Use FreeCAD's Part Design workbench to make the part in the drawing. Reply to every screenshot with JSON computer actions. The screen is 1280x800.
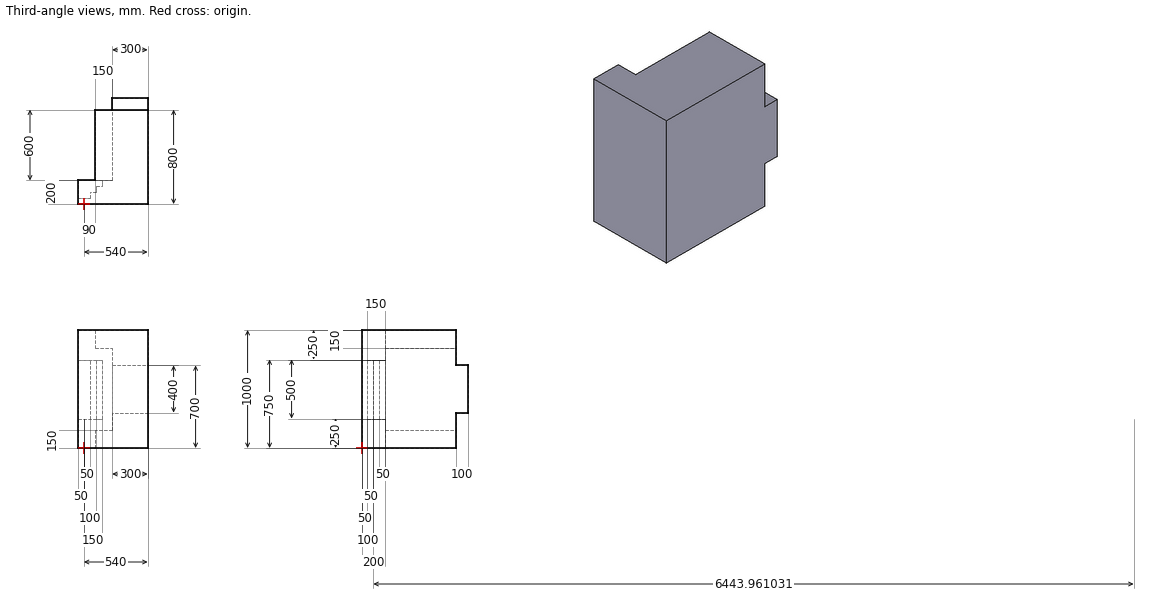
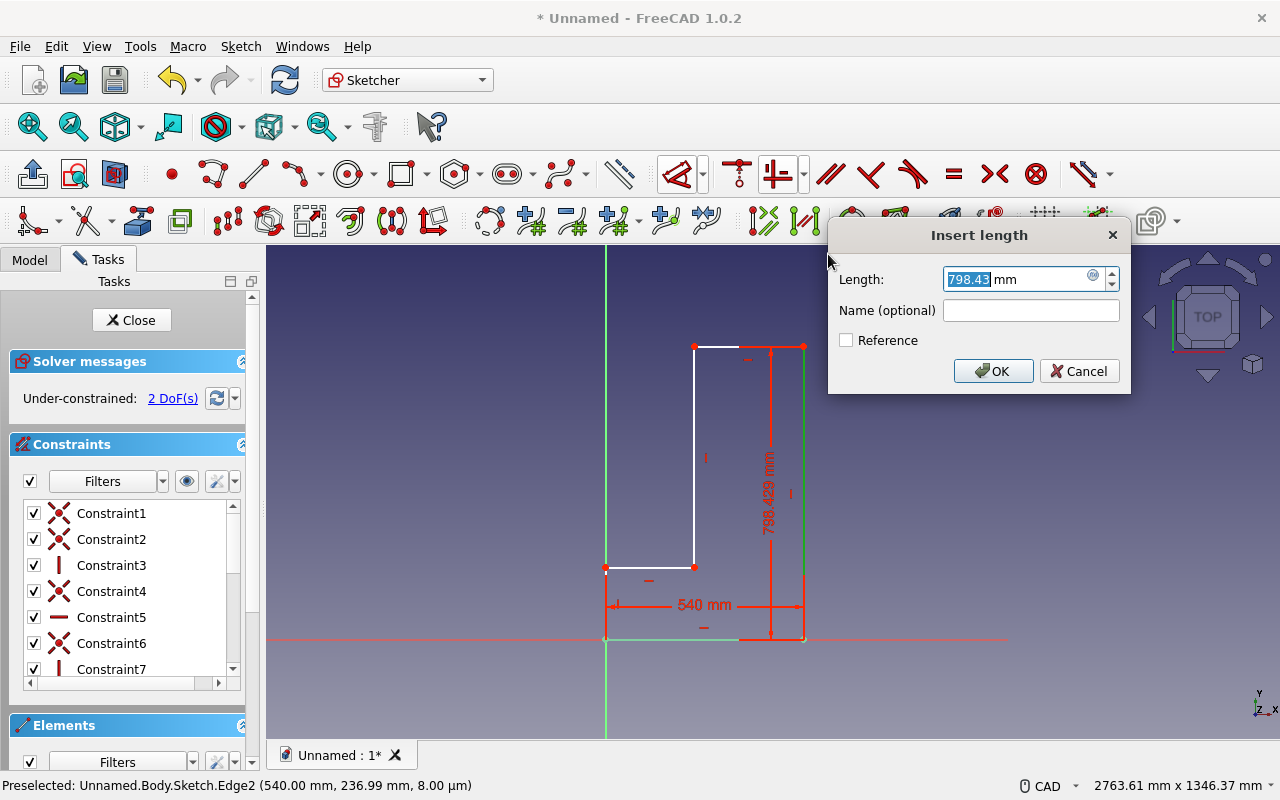
{"action": "type", "text": "800"}
{"action": "key", "text": "Return"}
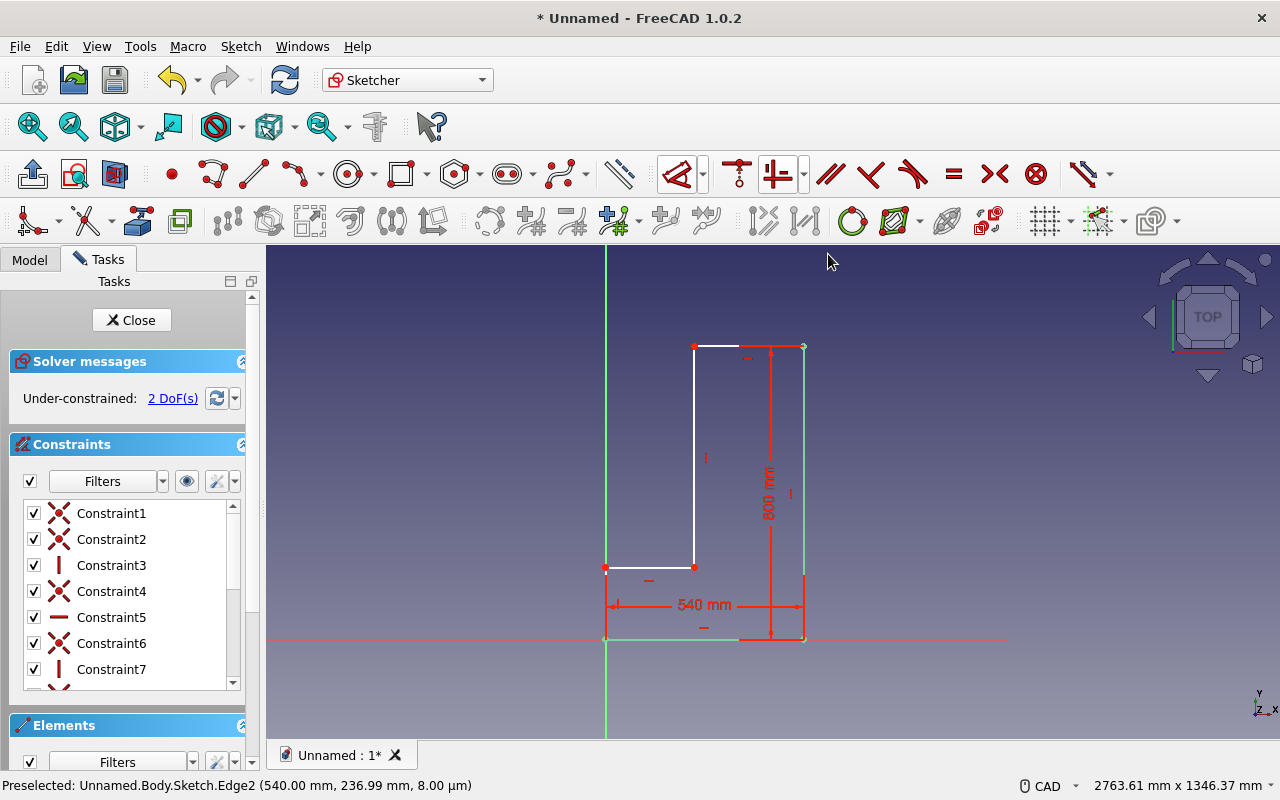
{"action": "left_click", "coordinate": [771, 346]}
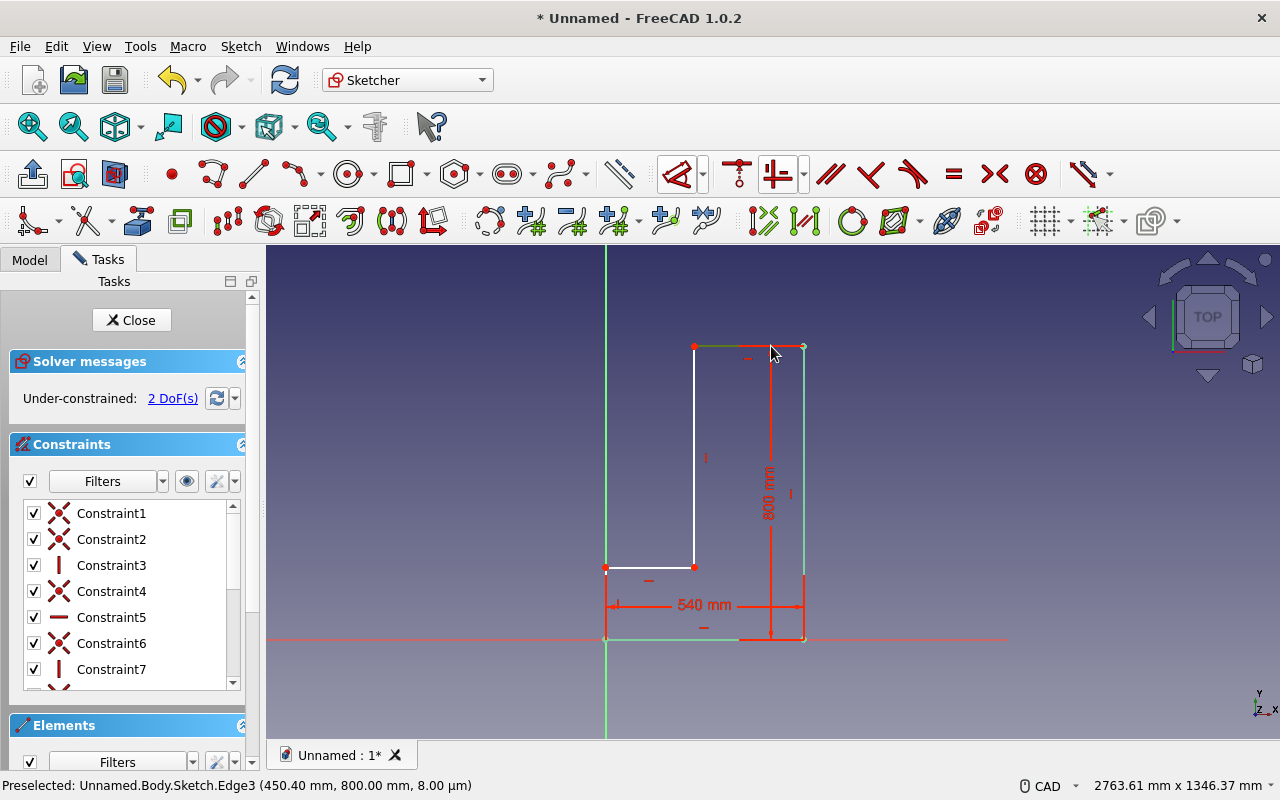
{"action": "key", "text": "l"}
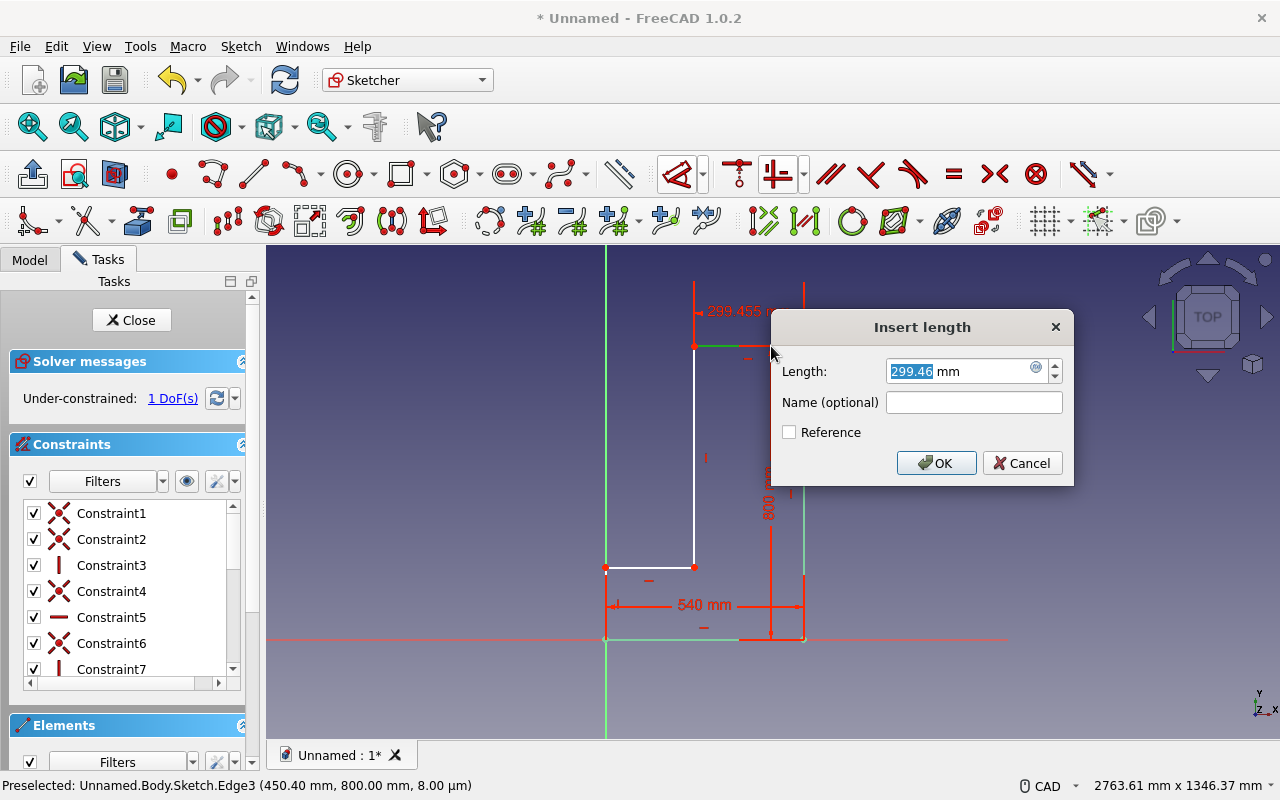
{"action": "type", "text": "300"}
{"action": "key", "text": "Return"}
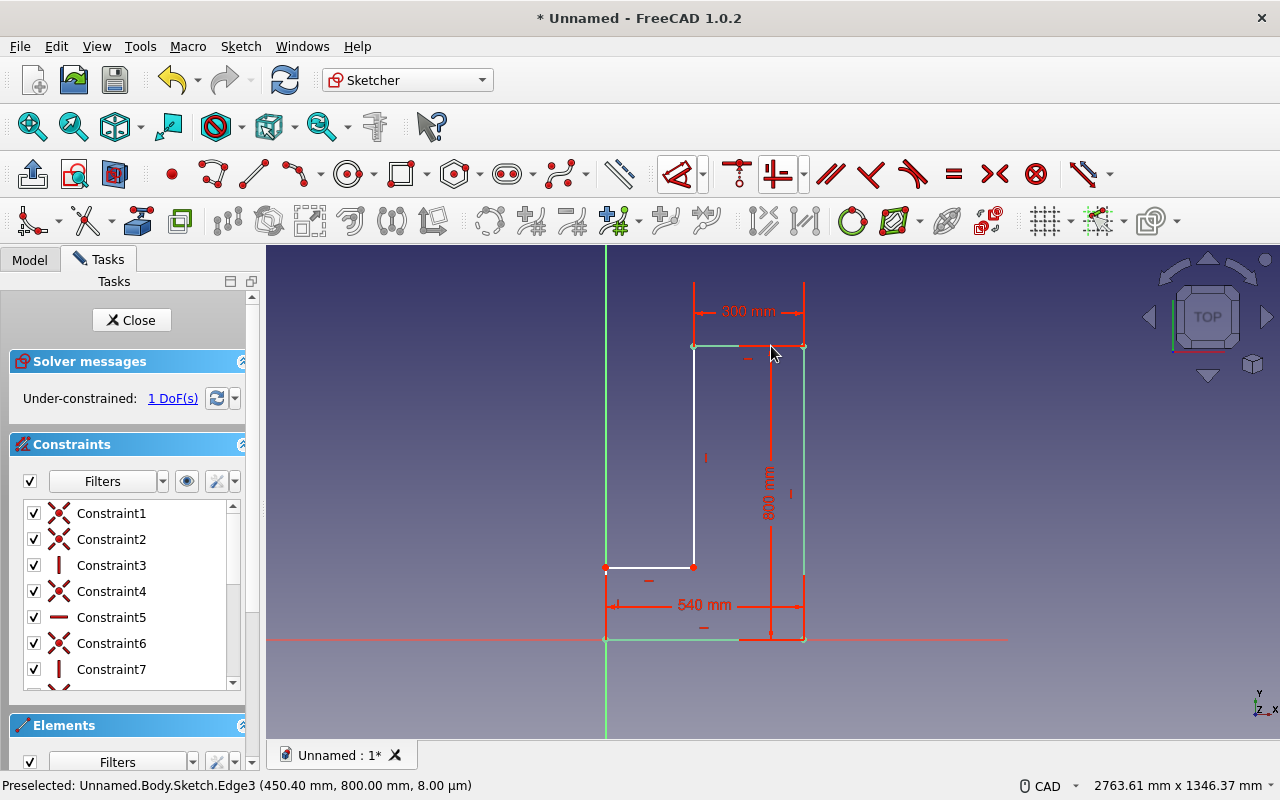
{"action": "left_click", "coordinate": [694, 413]}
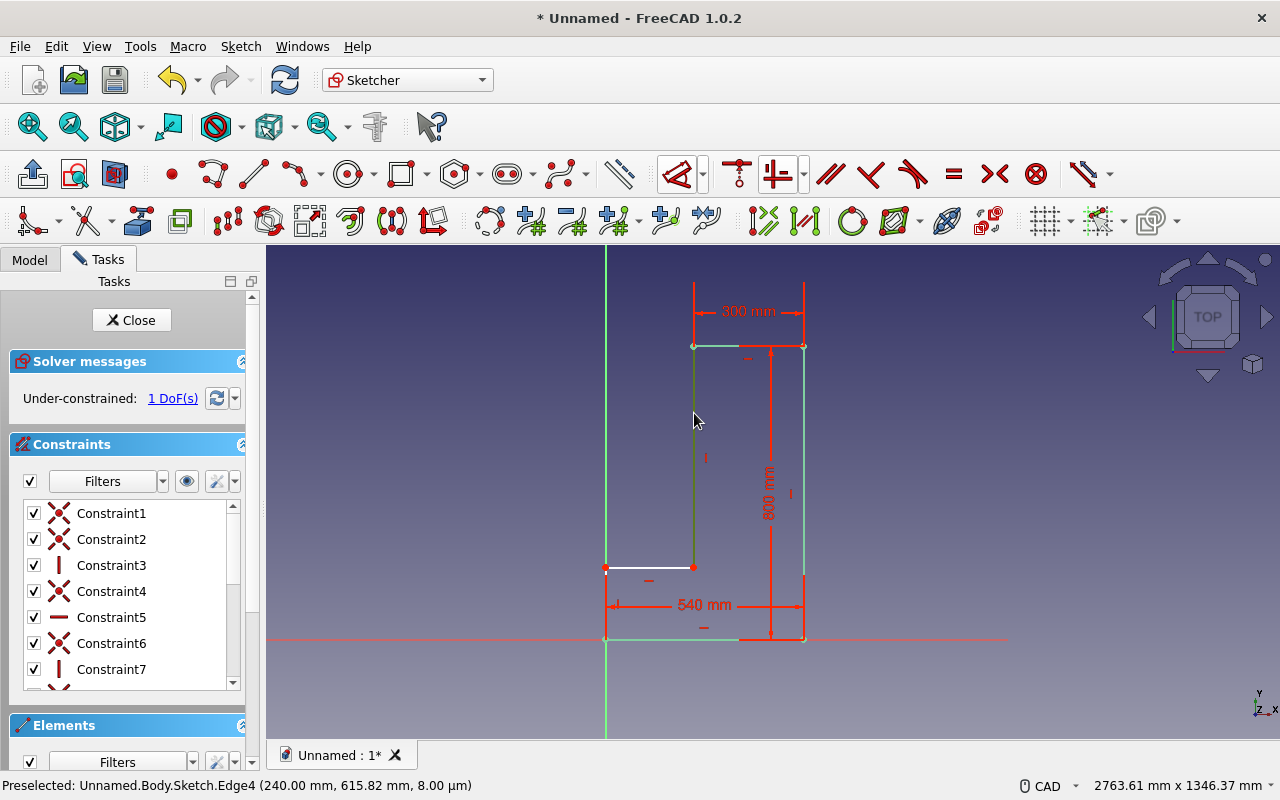
{"action": "key", "text": "i"}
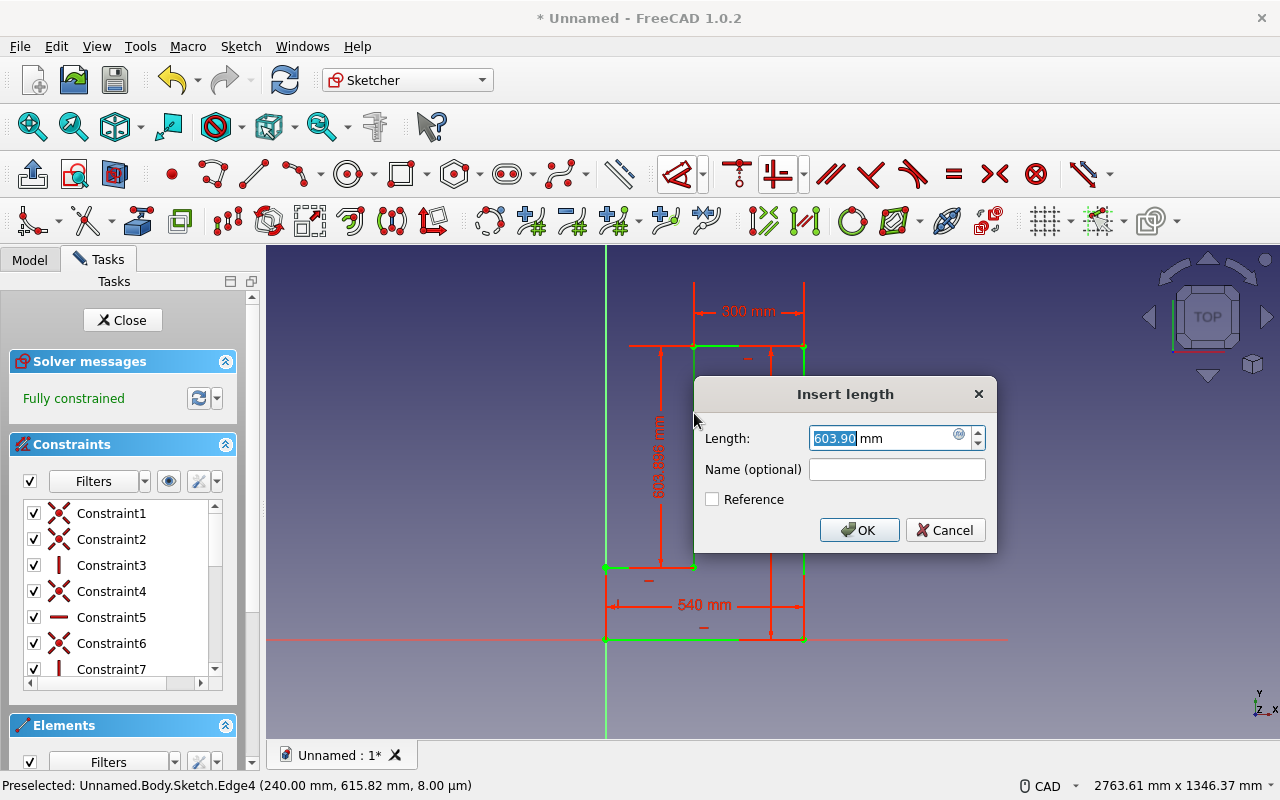
{"action": "type", "text": "600"}
{"action": "key", "text": "Return"}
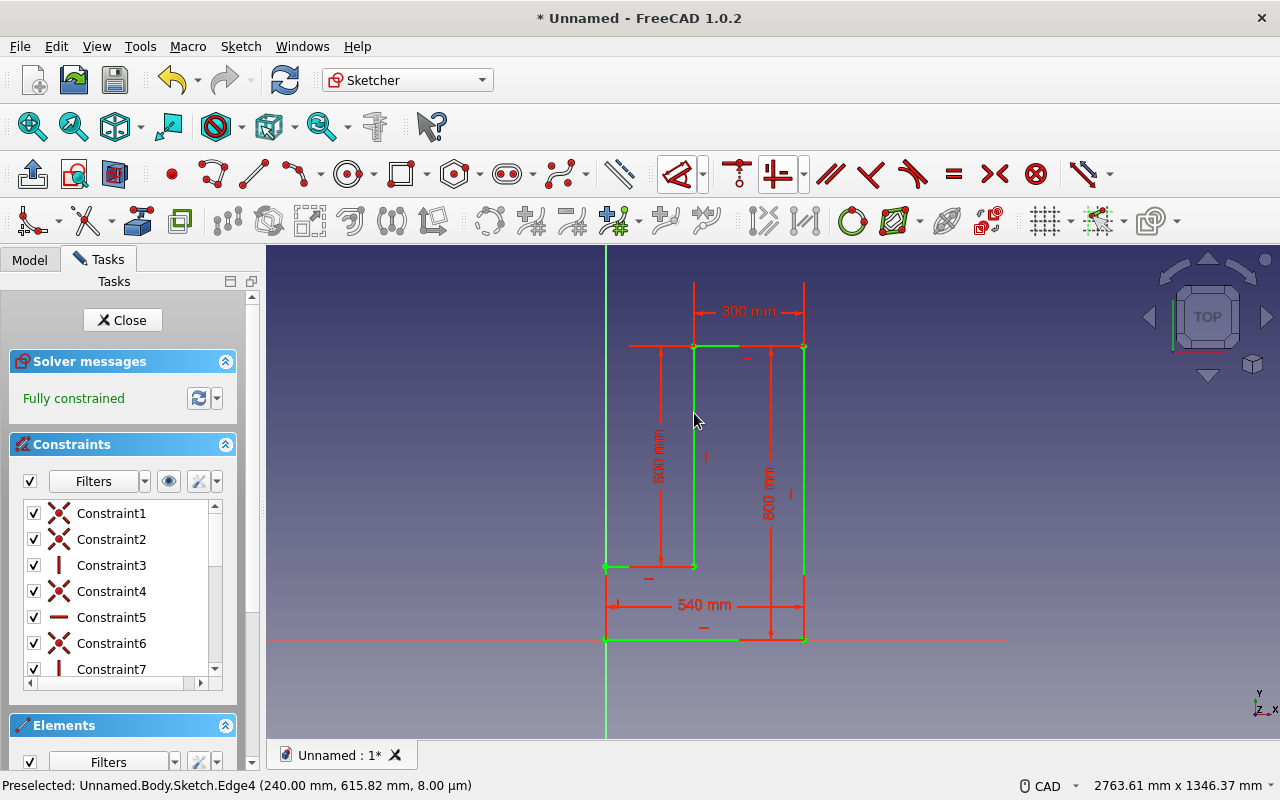
{"action": "left_click", "coordinate": [123, 320]}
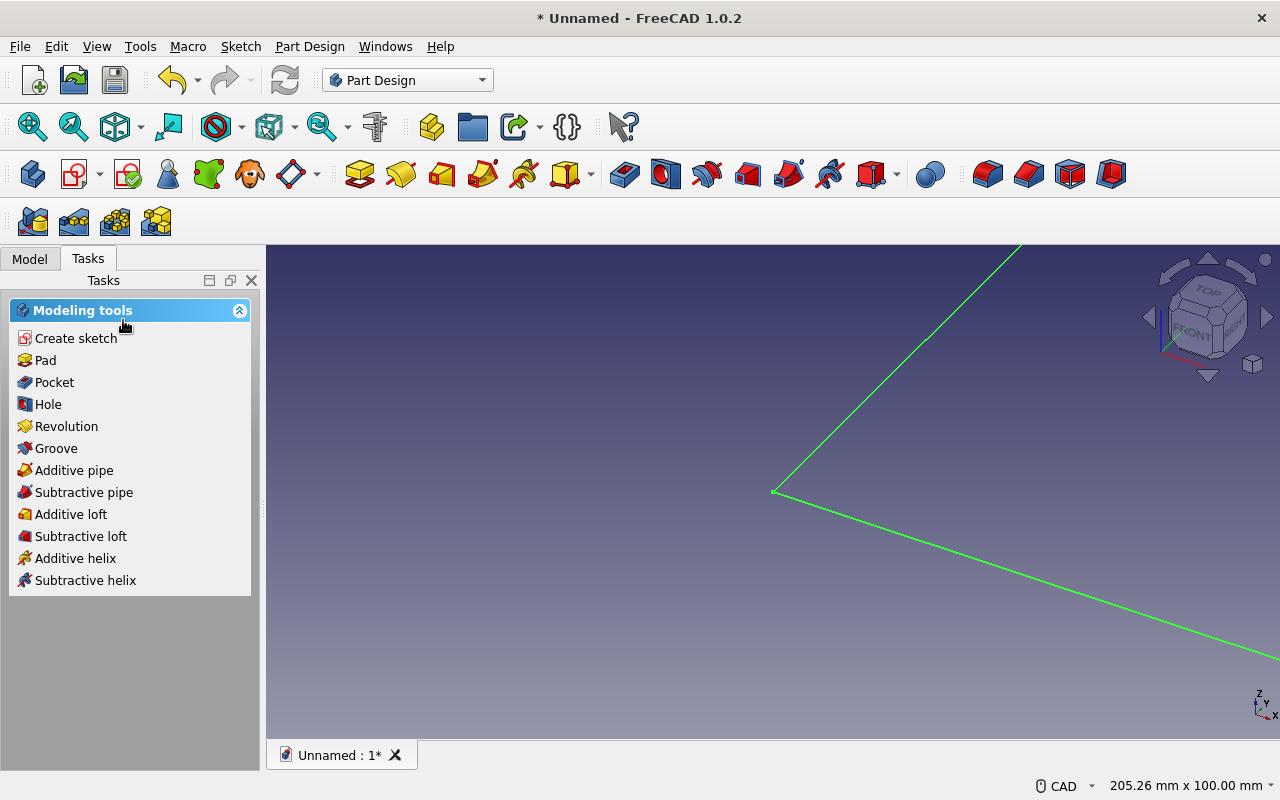
{"action": "left_click", "coordinate": [360, 174]}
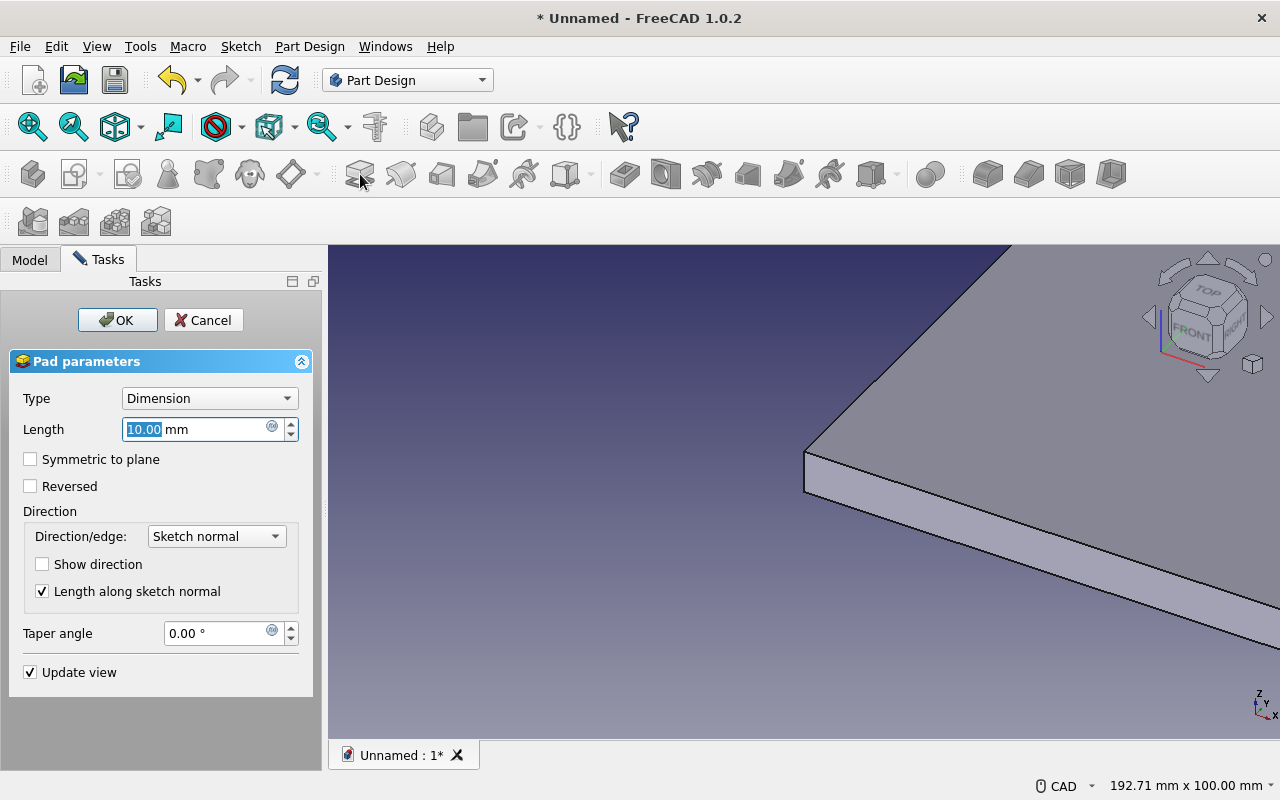
{"action": "type", "text": "1000"}
{"action": "key", "text": "Tab"}